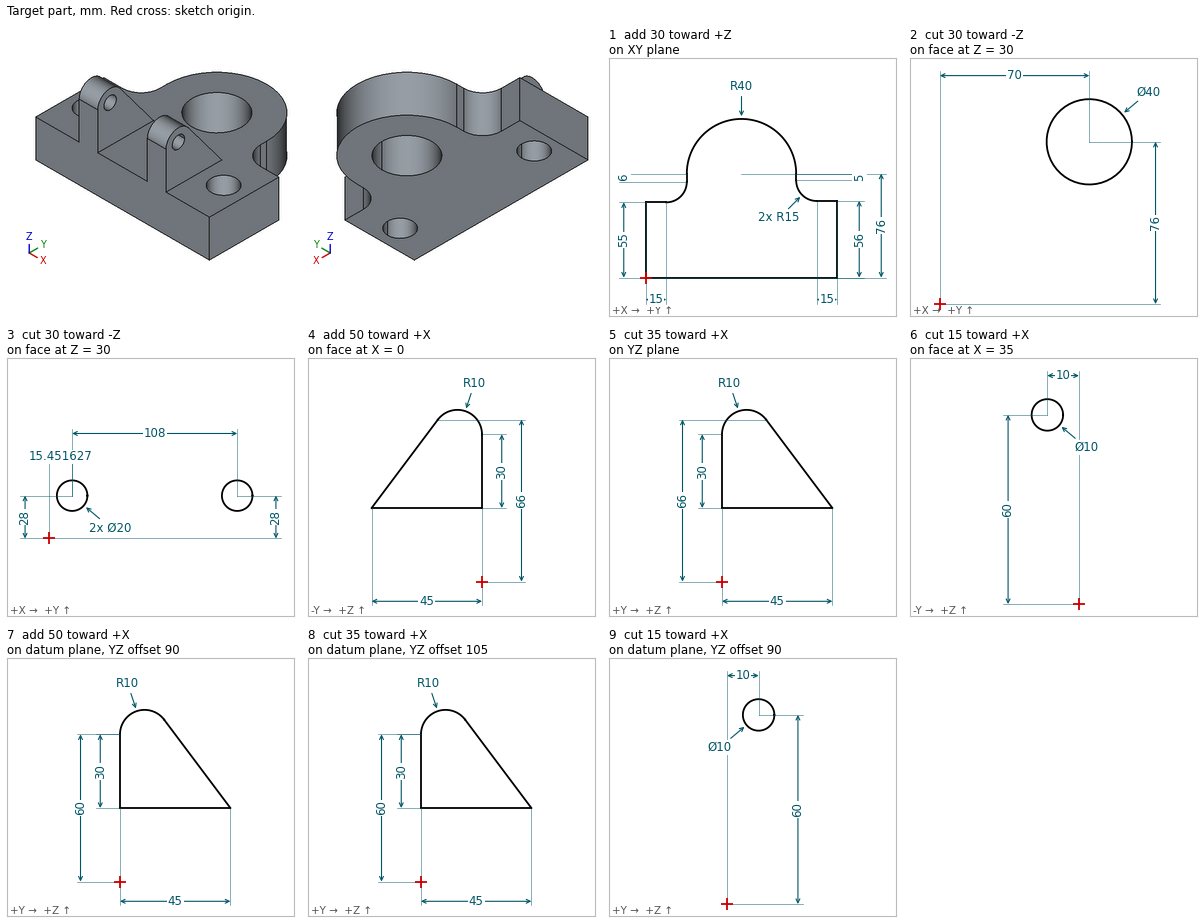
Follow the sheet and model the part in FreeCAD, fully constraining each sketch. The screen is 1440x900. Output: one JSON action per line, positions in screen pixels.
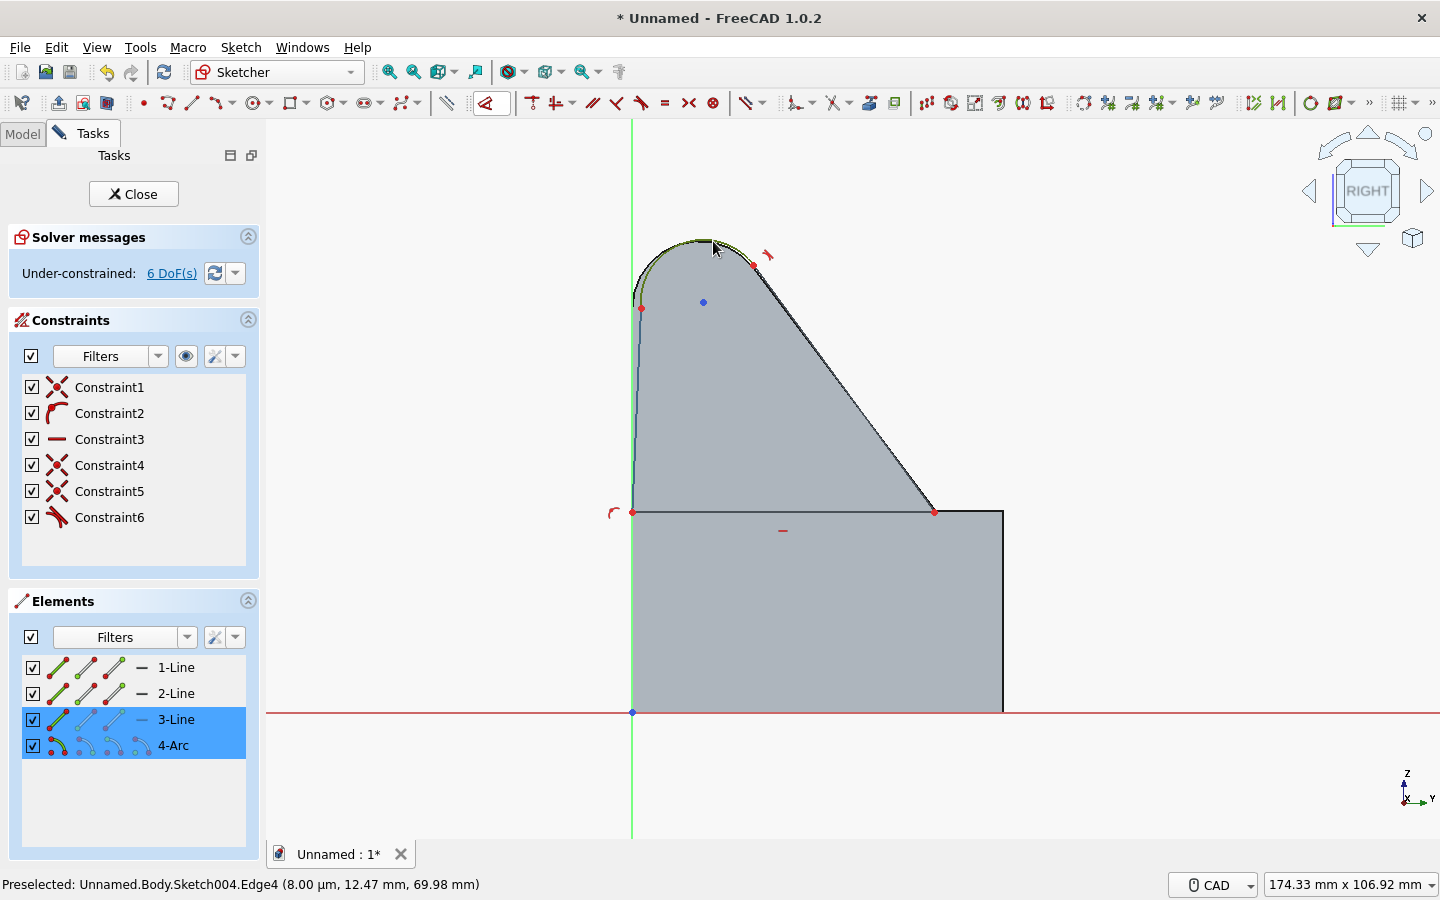
{"action": "key", "text": "t"}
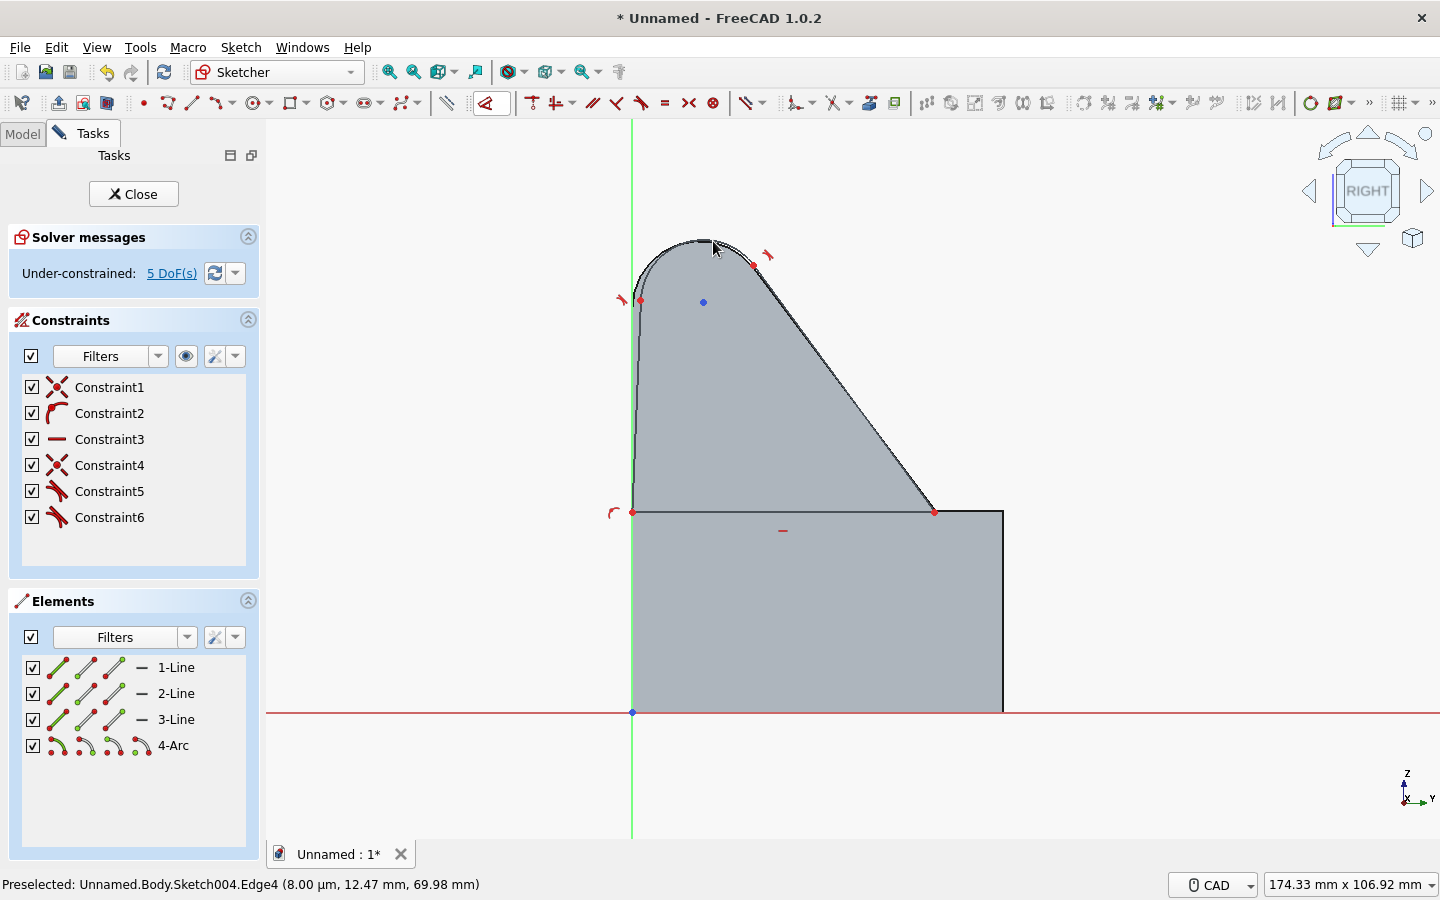
{"action": "left_click", "coordinate": [635, 448]}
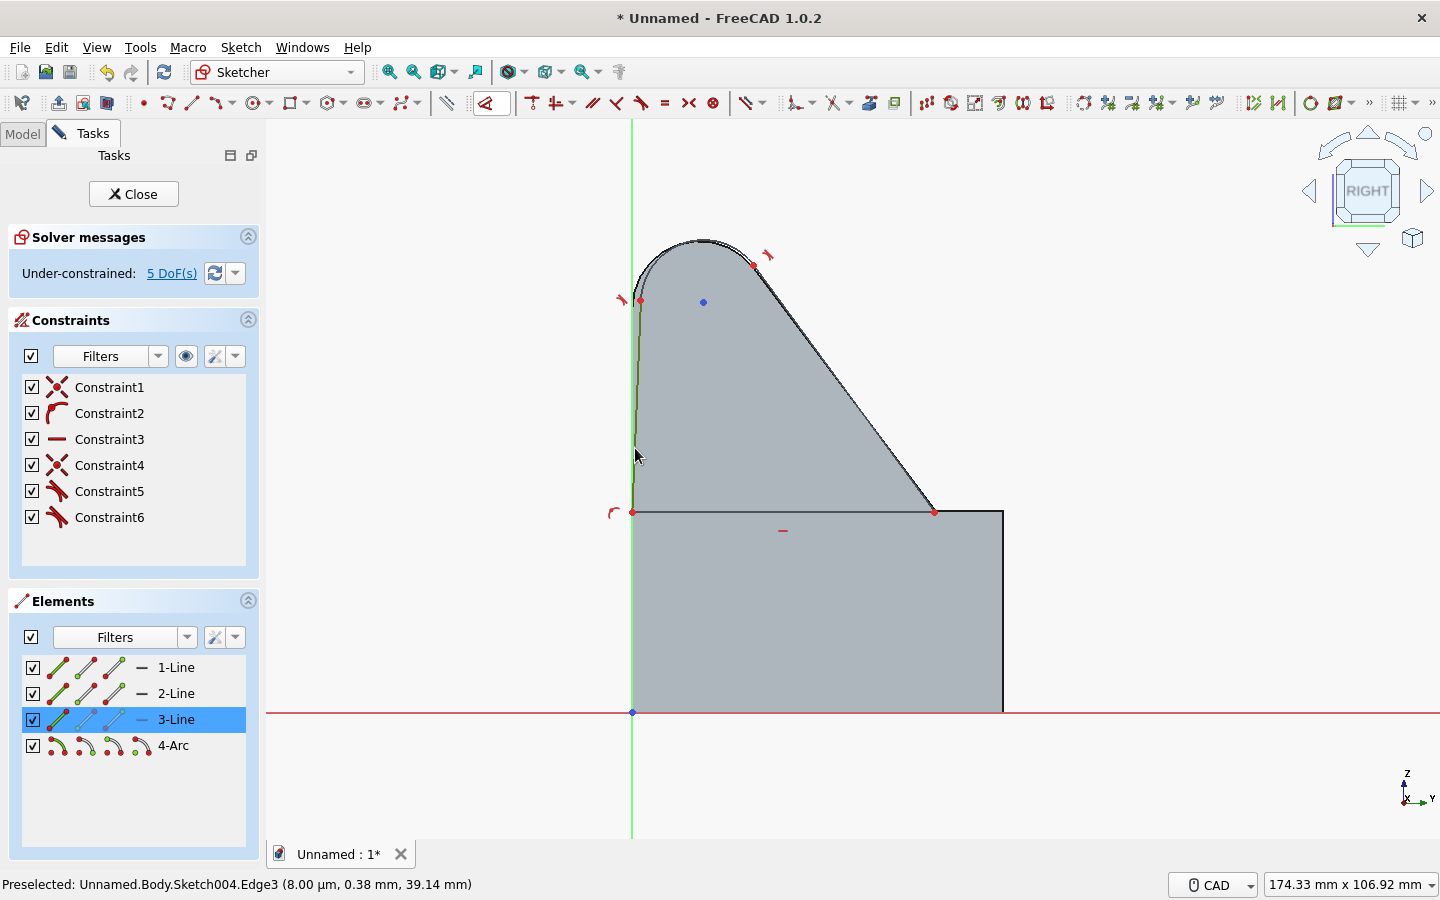
{"action": "key", "text": "v"}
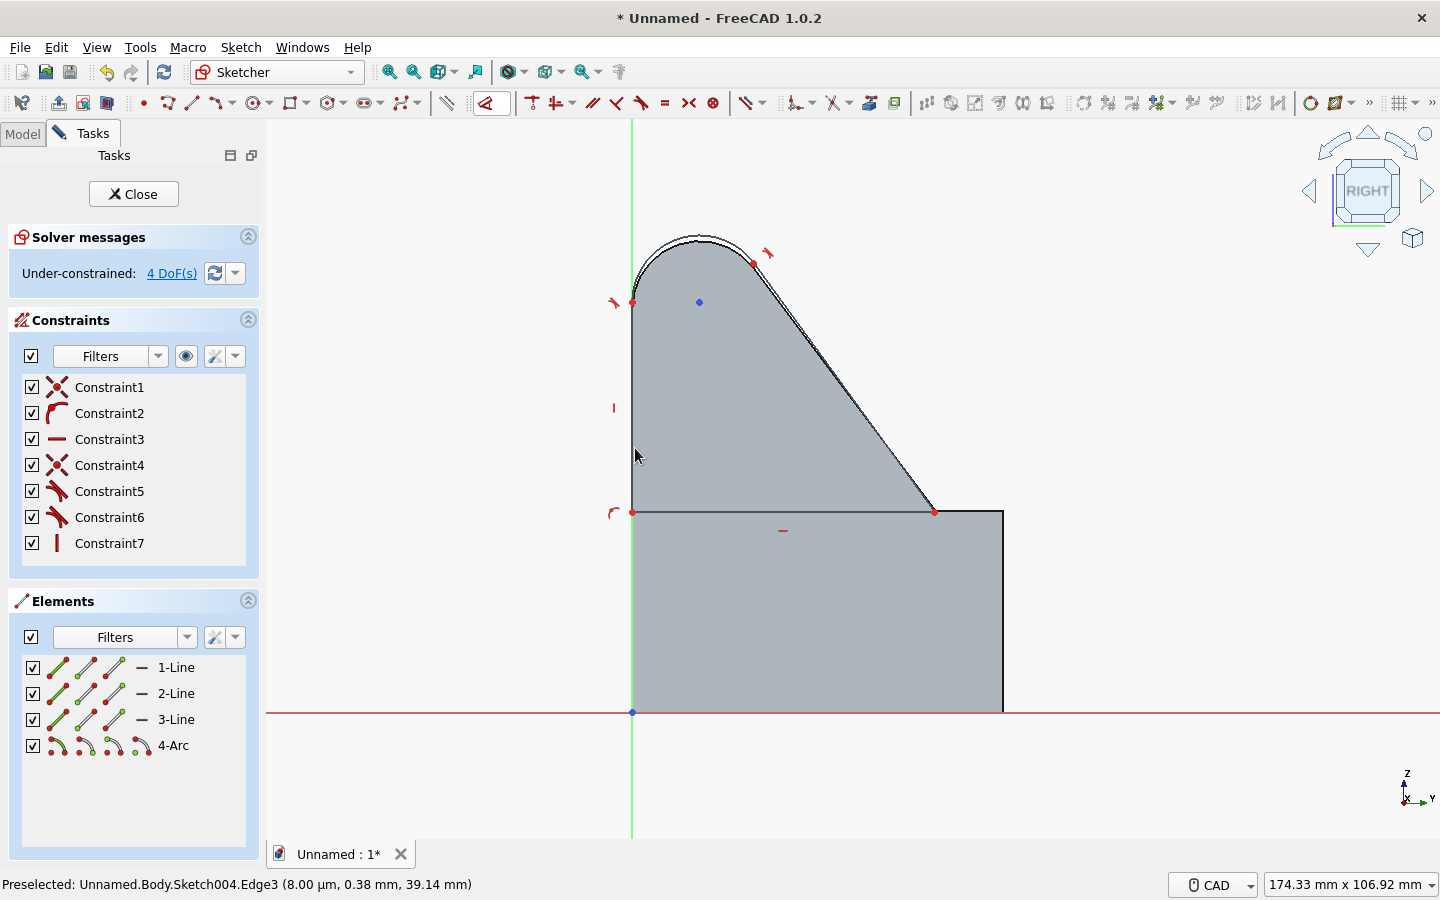
{"action": "left_click", "coordinate": [712, 237]}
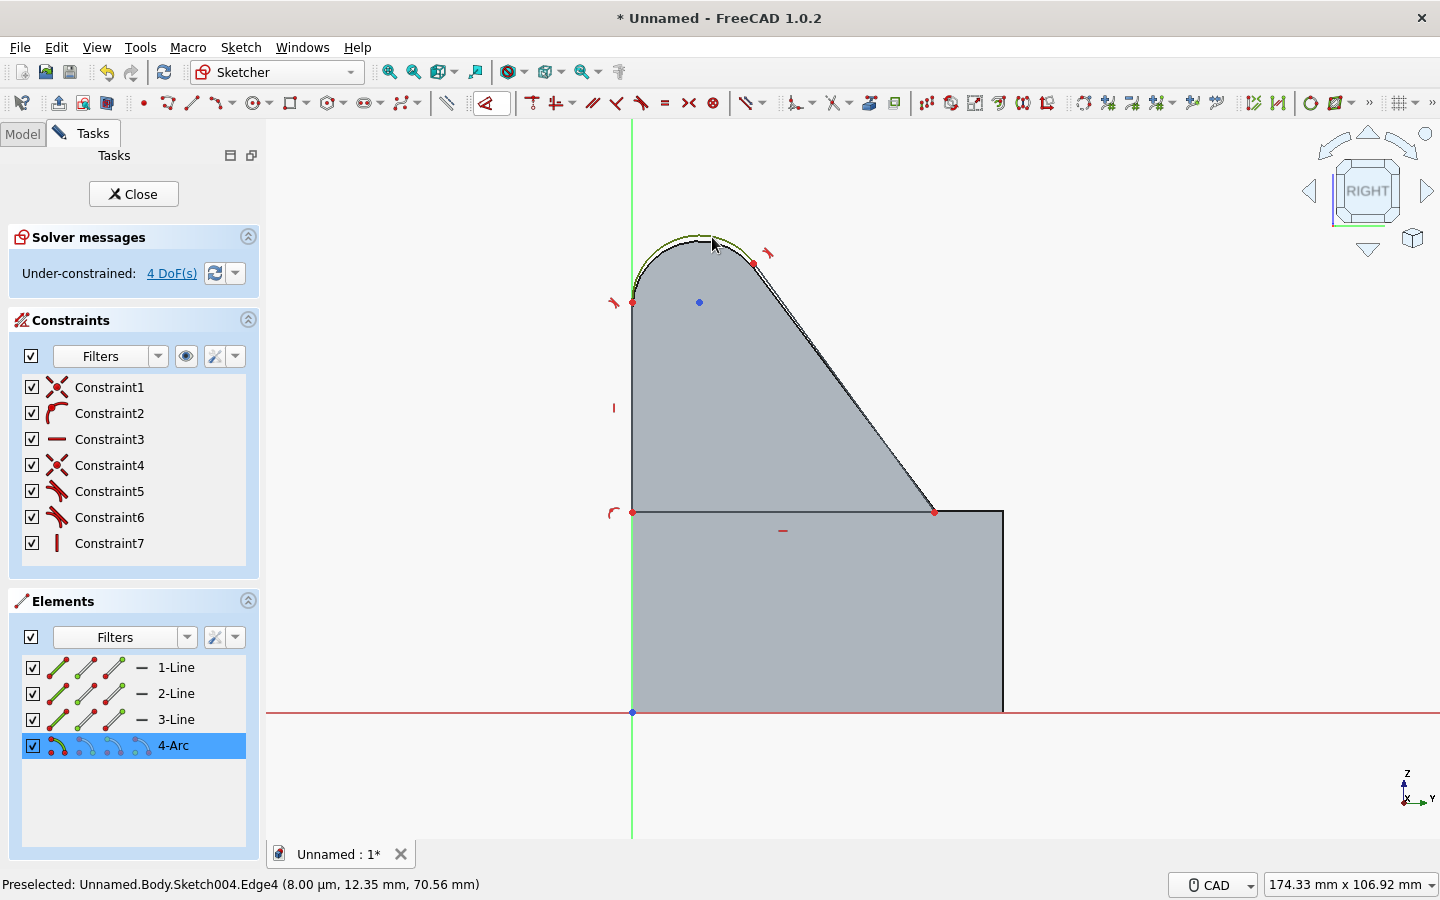
{"action": "left_click", "coordinate": [504, 104]}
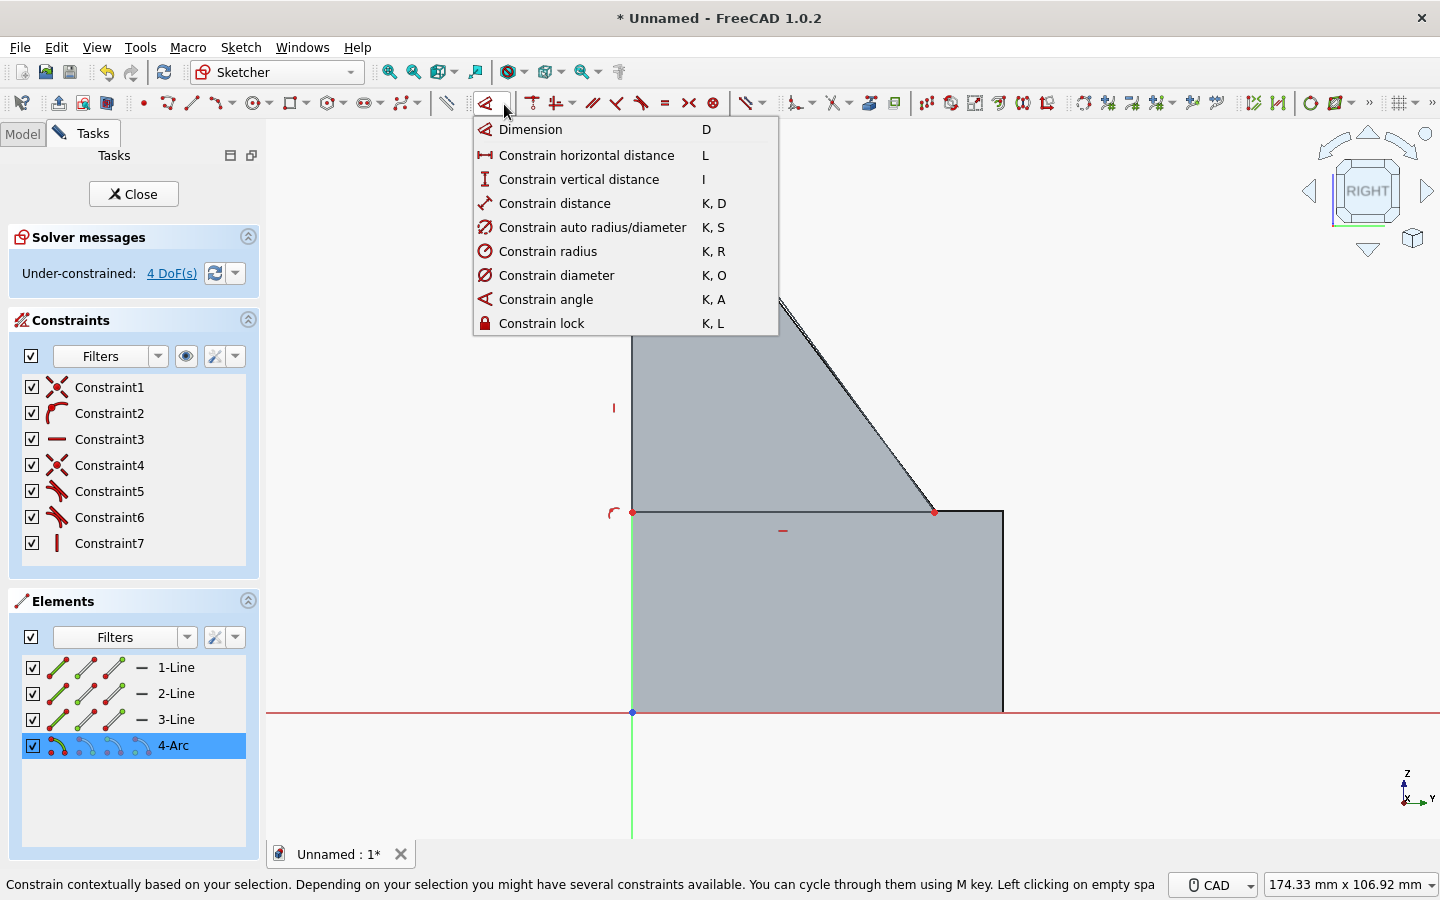
{"action": "left_click", "coordinate": [626, 251]}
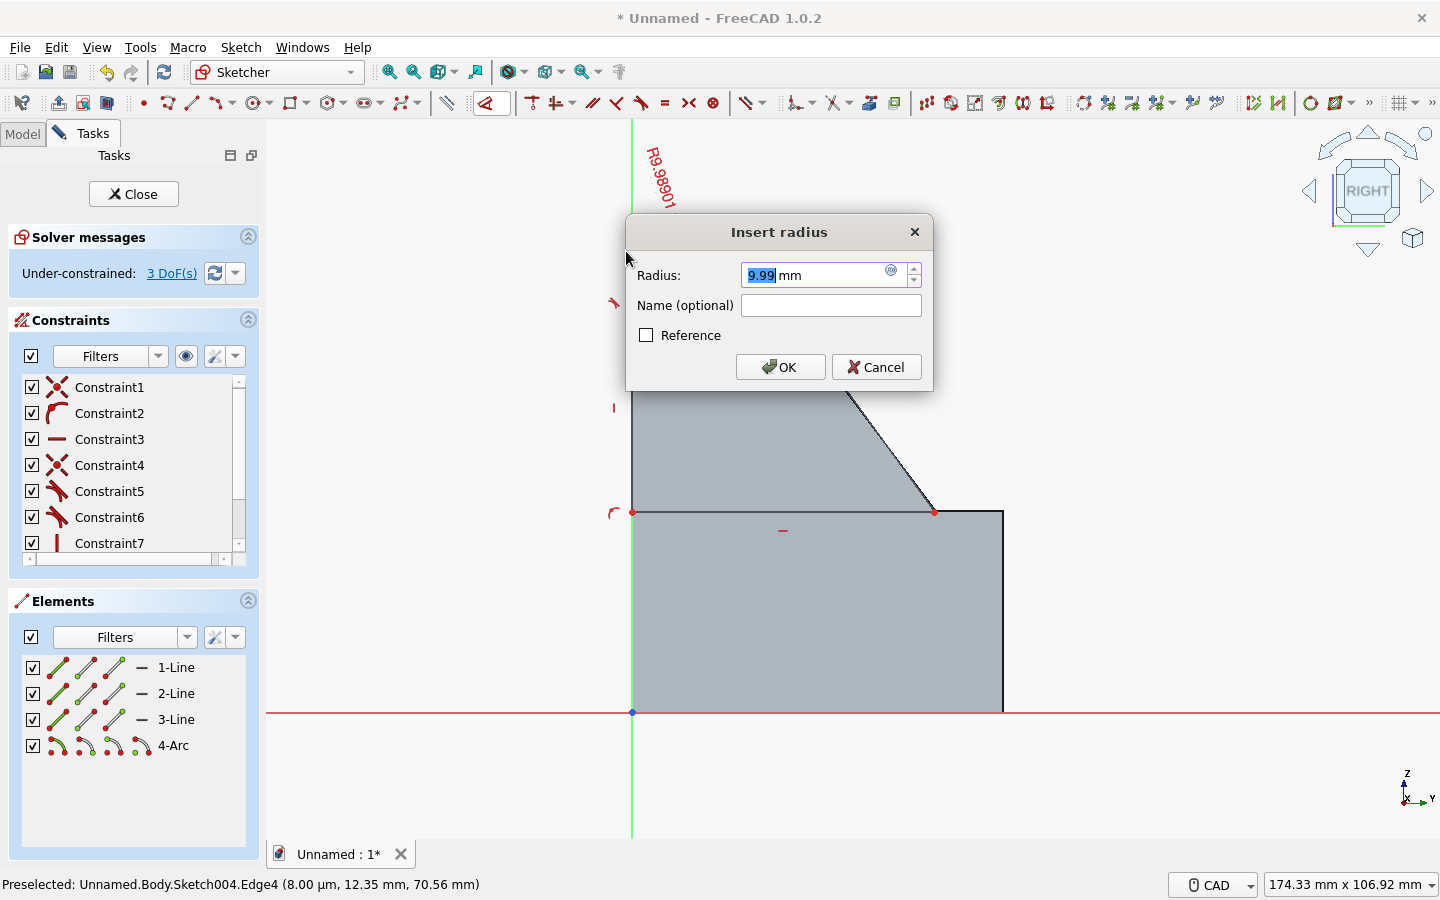
{"action": "type", "text": "10"}
{"action": "key", "text": "Return"}